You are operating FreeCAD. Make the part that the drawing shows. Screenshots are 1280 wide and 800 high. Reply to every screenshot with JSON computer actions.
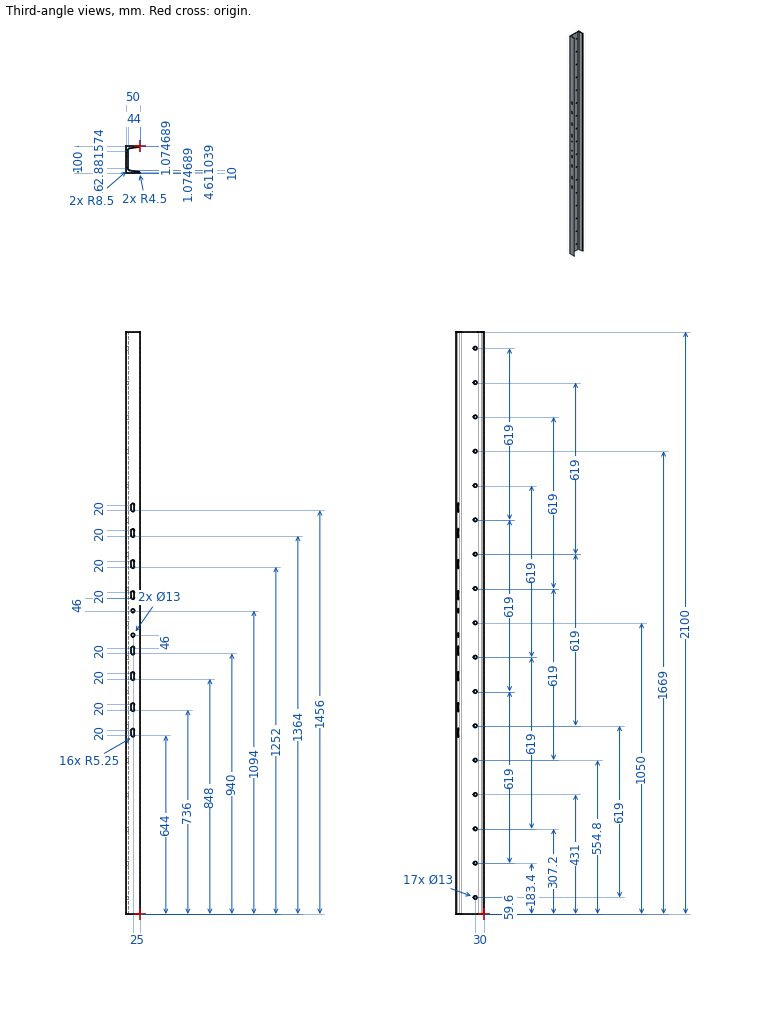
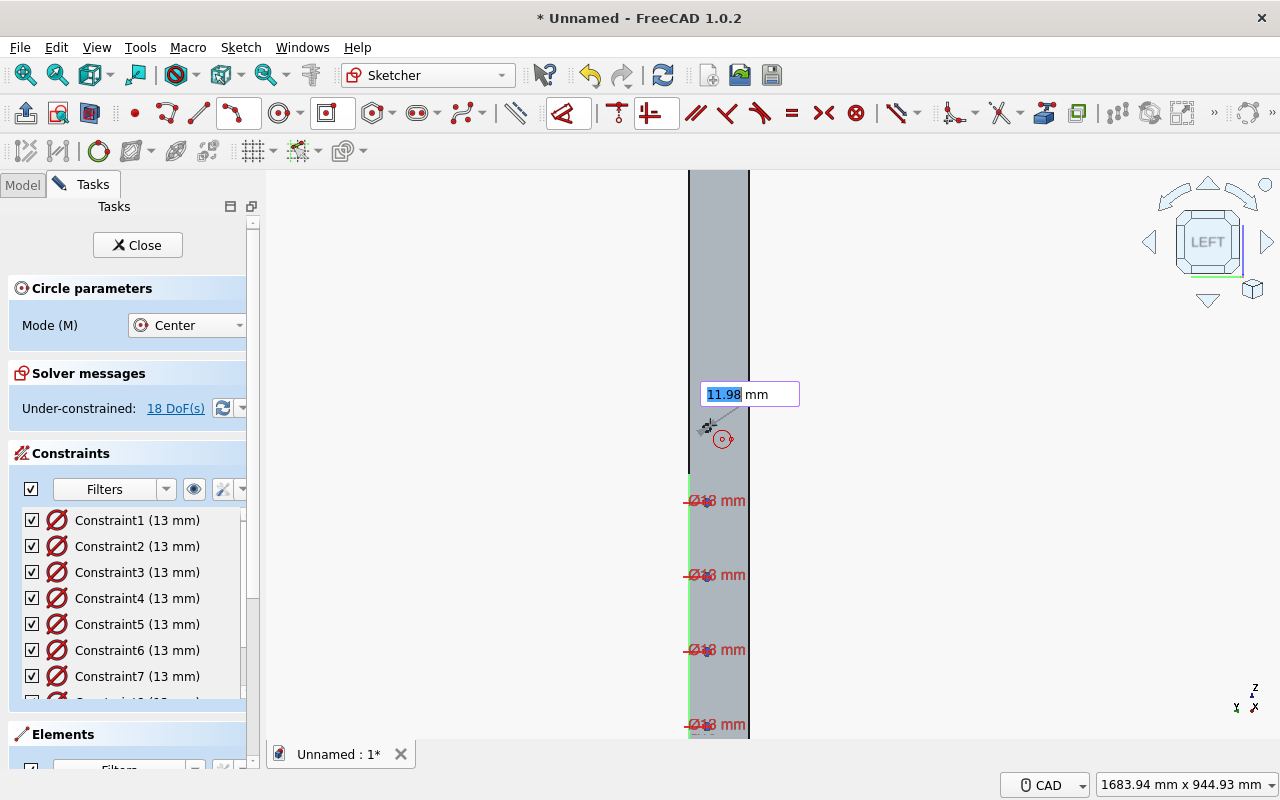
{"action": "type", "text": "13"}
{"action": "key", "text": "Return"}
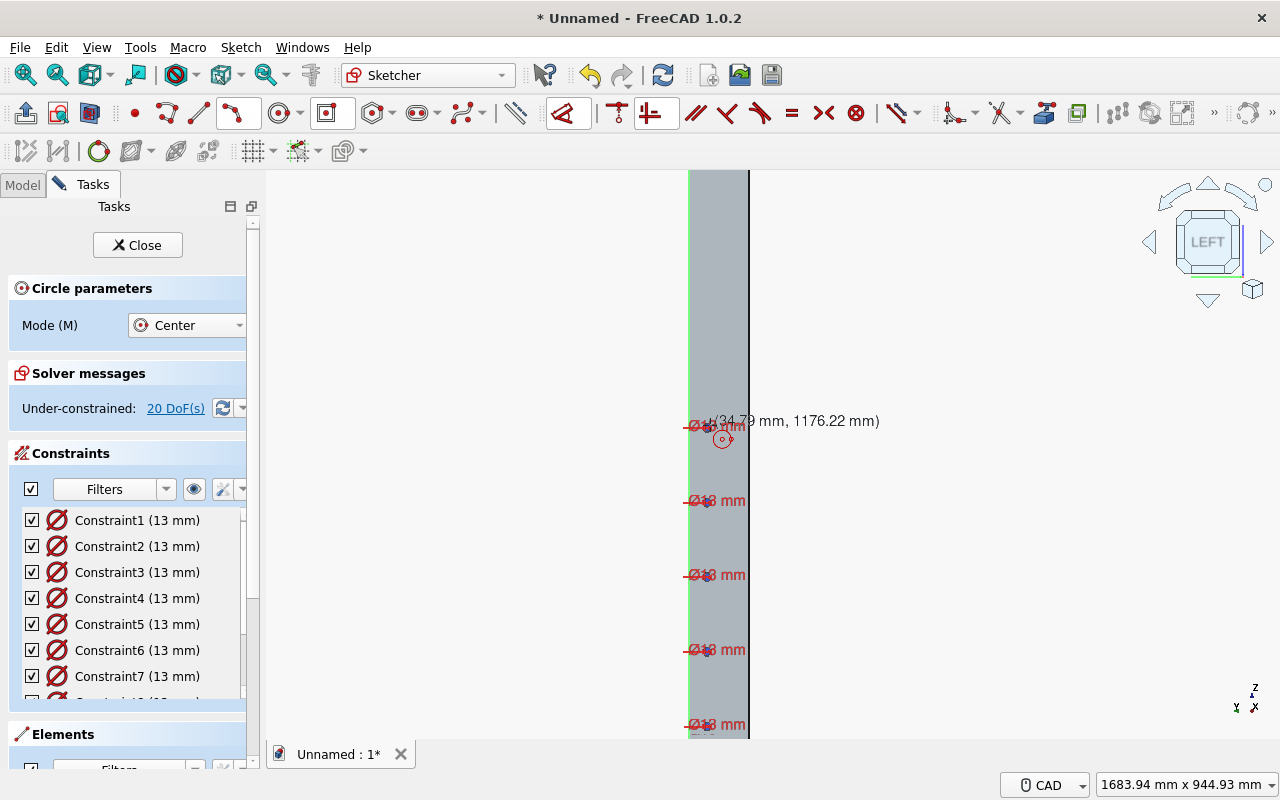
{"action": "scroll", "coordinate": [707, 353], "scroll_direction": "up", "scroll_amount": 9}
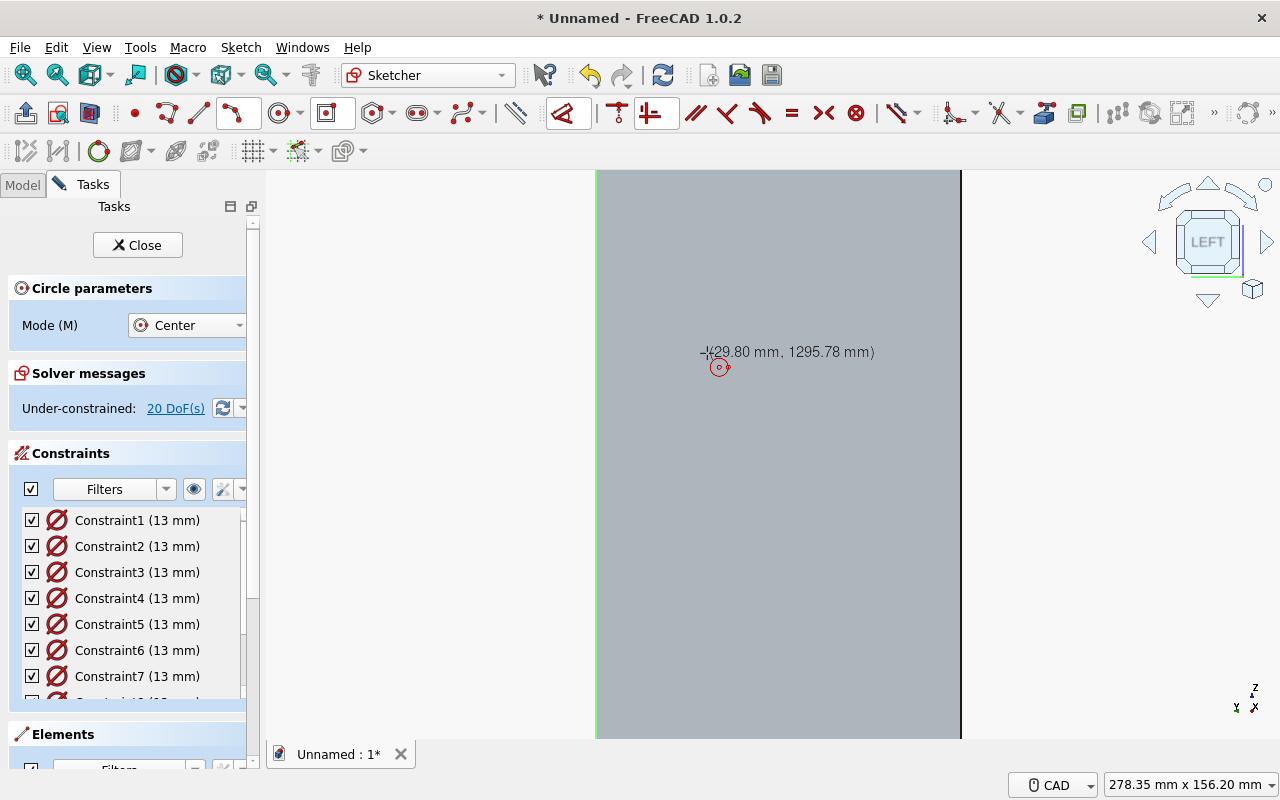
{"action": "scroll", "coordinate": [707, 408], "scroll_direction": "down", "scroll_amount": 15}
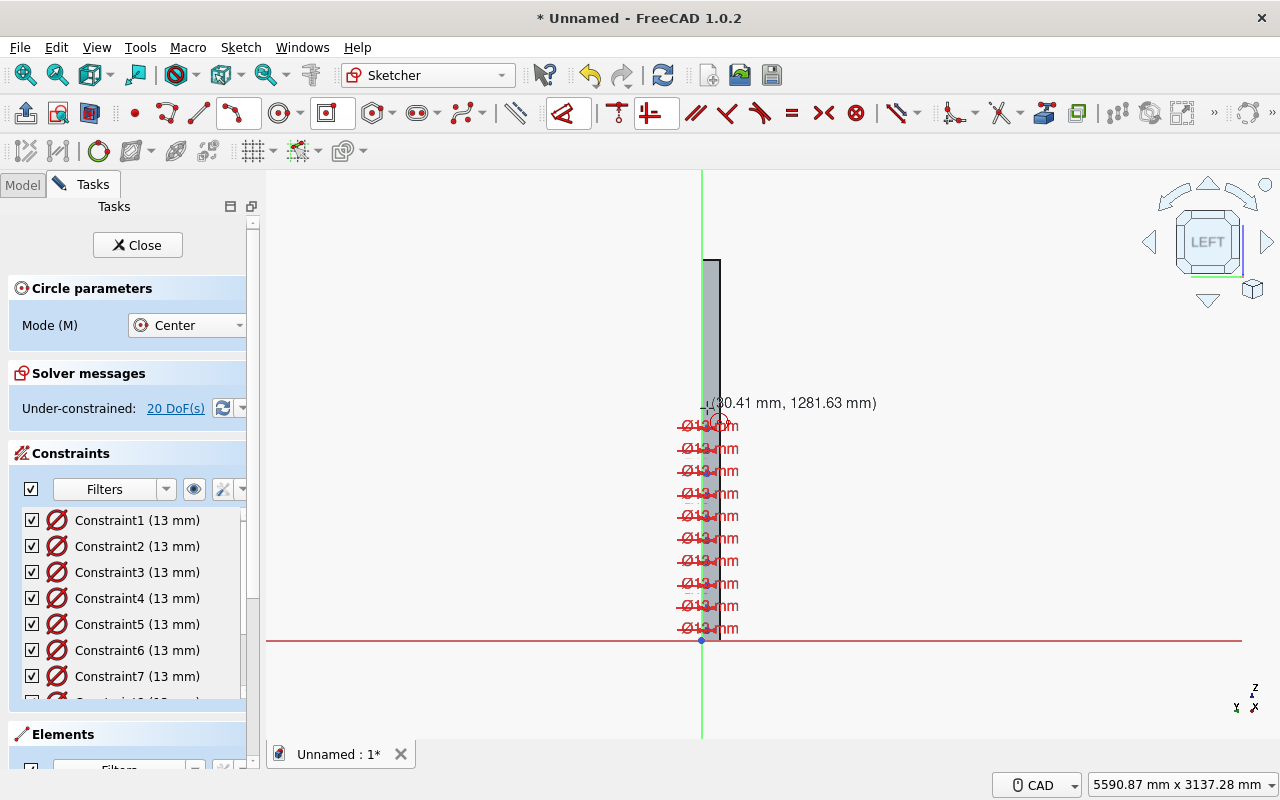
{"action": "scroll", "coordinate": [707, 406], "scroll_direction": "up", "scroll_amount": 6}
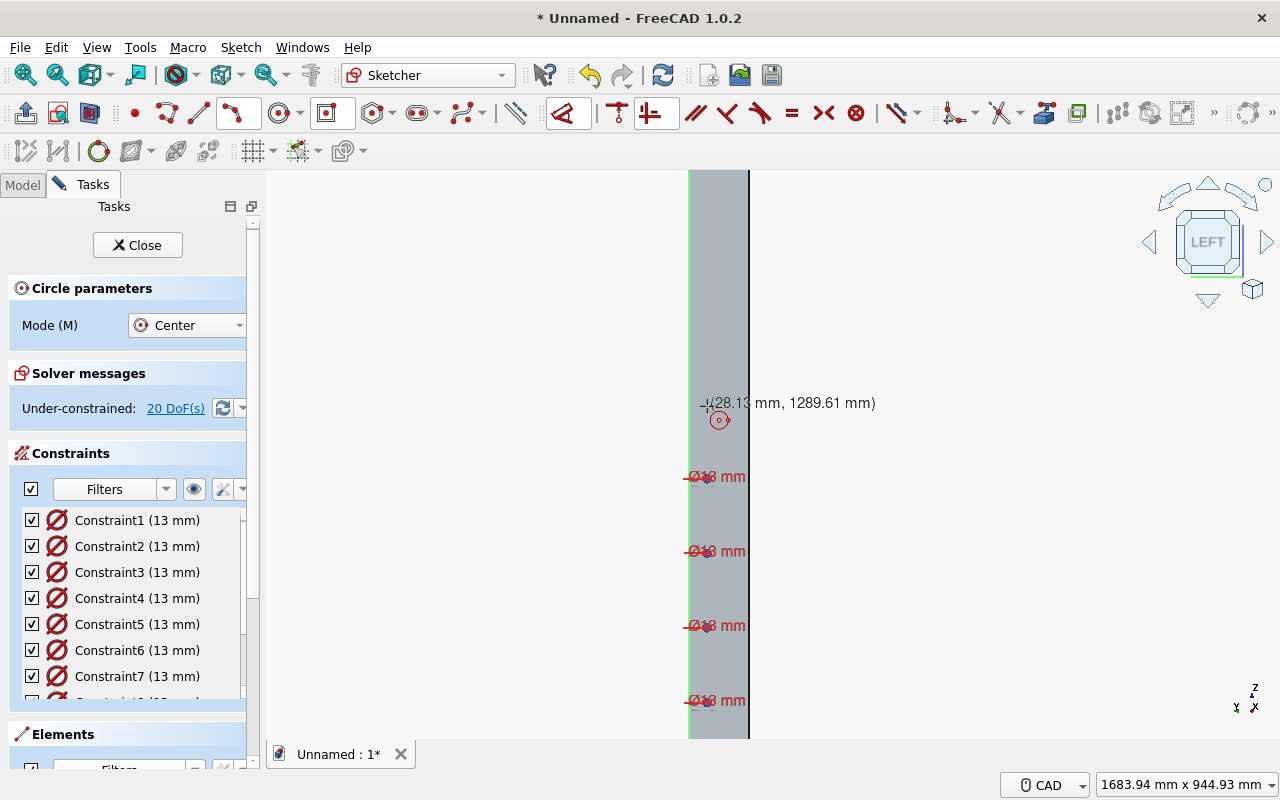
{"action": "left_click", "coordinate": [707, 404]}
{"action": "mouse_move", "coordinate": [710, 401]}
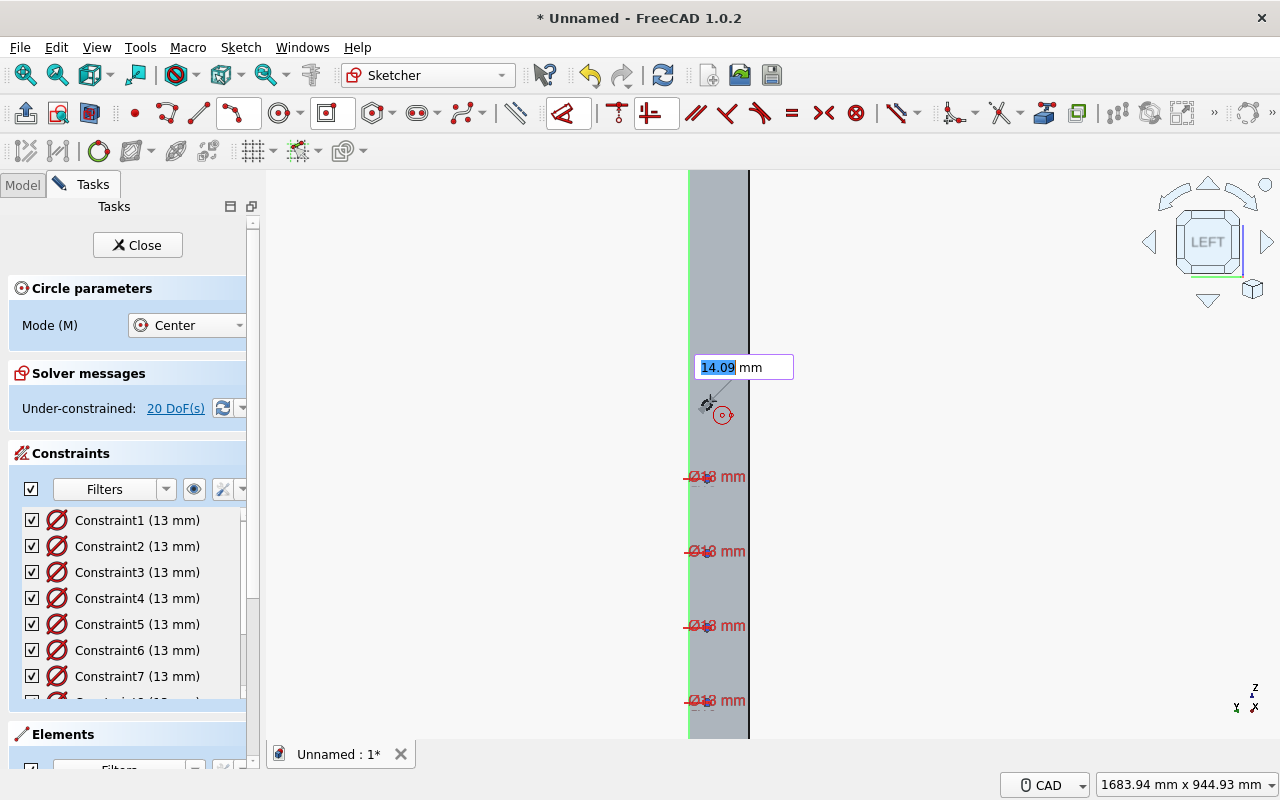
{"action": "type", "text": "13"}
{"action": "key", "text": "Return"}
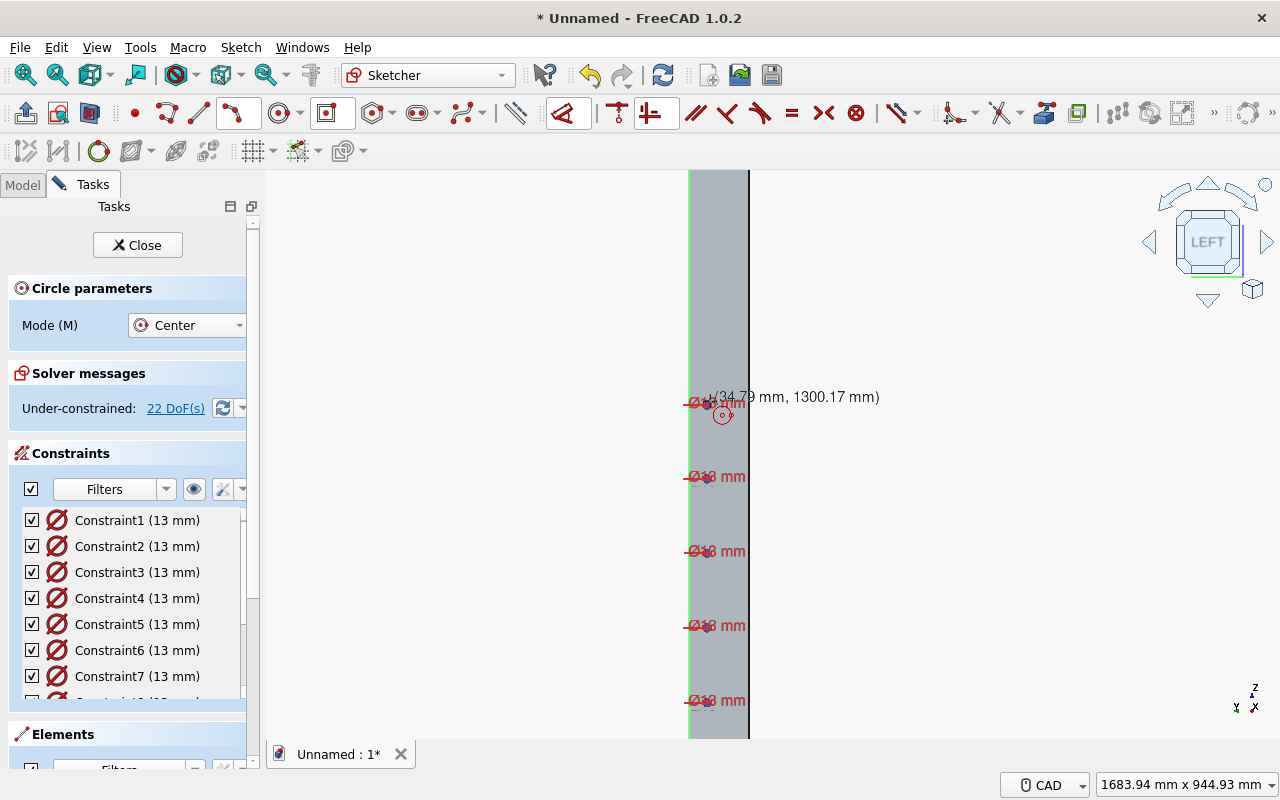
{"action": "scroll", "coordinate": [707, 329], "scroll_direction": "up", "scroll_amount": 9}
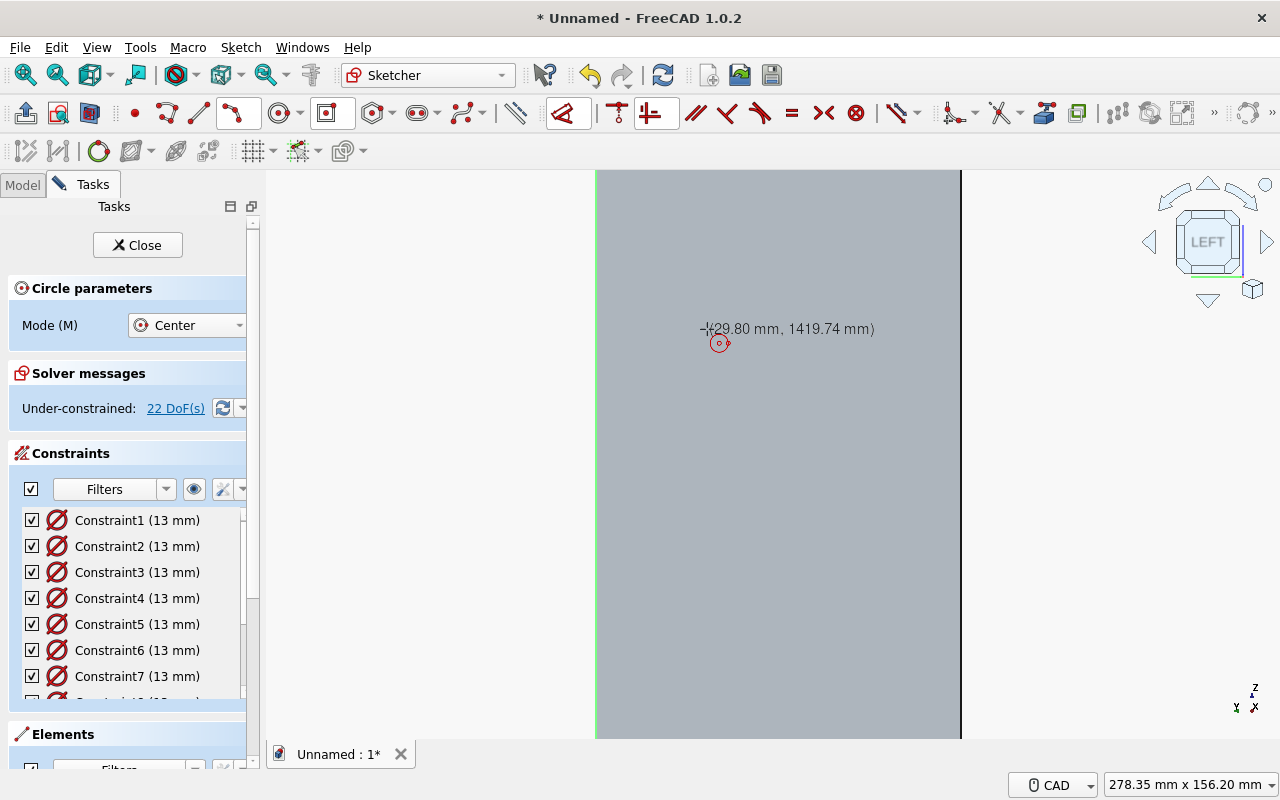
{"action": "scroll", "coordinate": [707, 385], "scroll_direction": "down", "scroll_amount": 15}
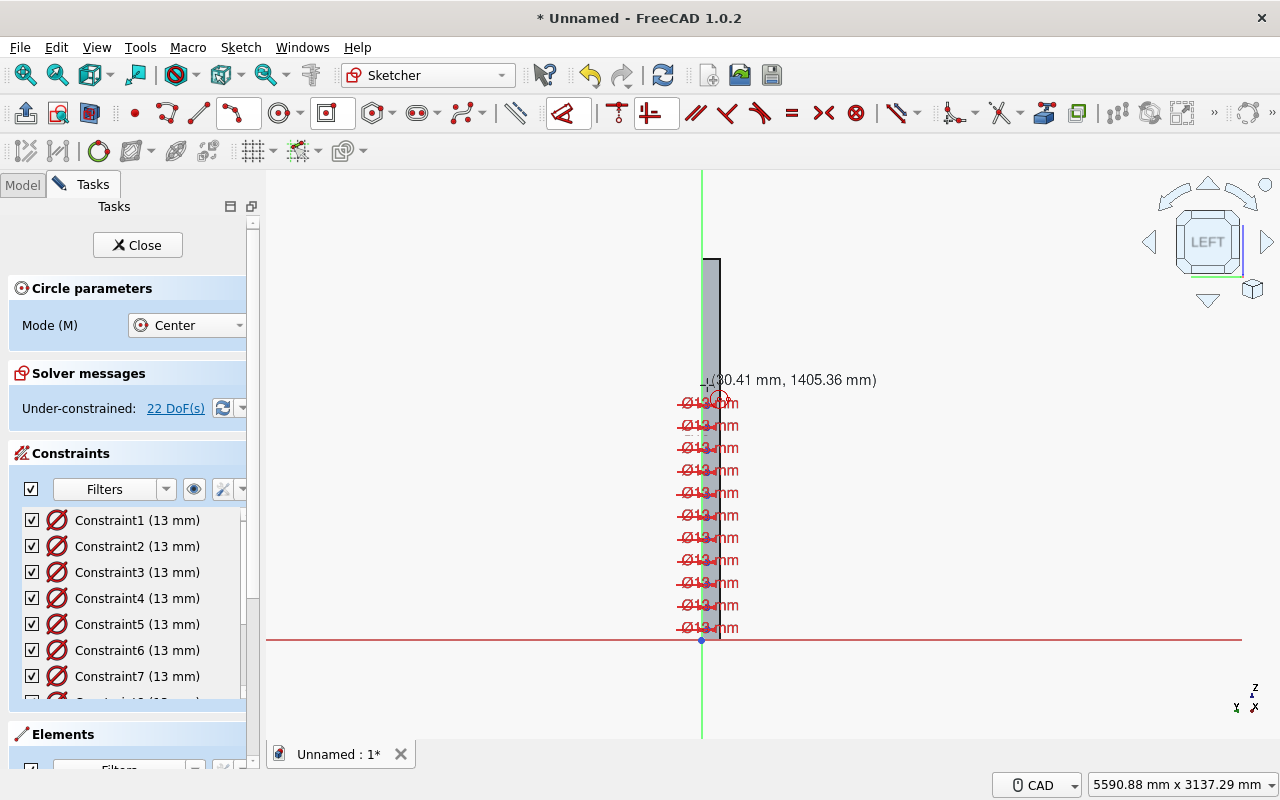
{"action": "scroll", "coordinate": [707, 383], "scroll_direction": "up", "scroll_amount": 6}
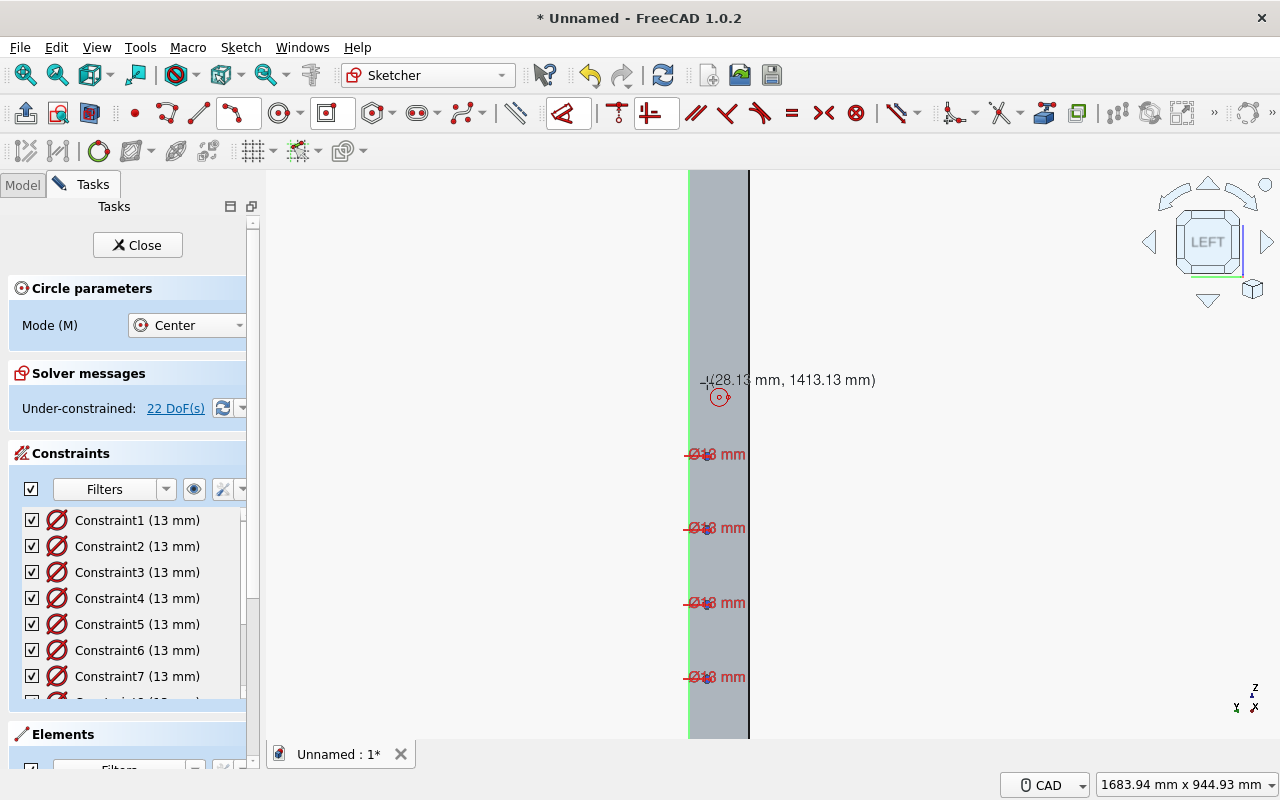
{"action": "left_click", "coordinate": [707, 380]}
{"action": "mouse_move", "coordinate": [710, 378]}